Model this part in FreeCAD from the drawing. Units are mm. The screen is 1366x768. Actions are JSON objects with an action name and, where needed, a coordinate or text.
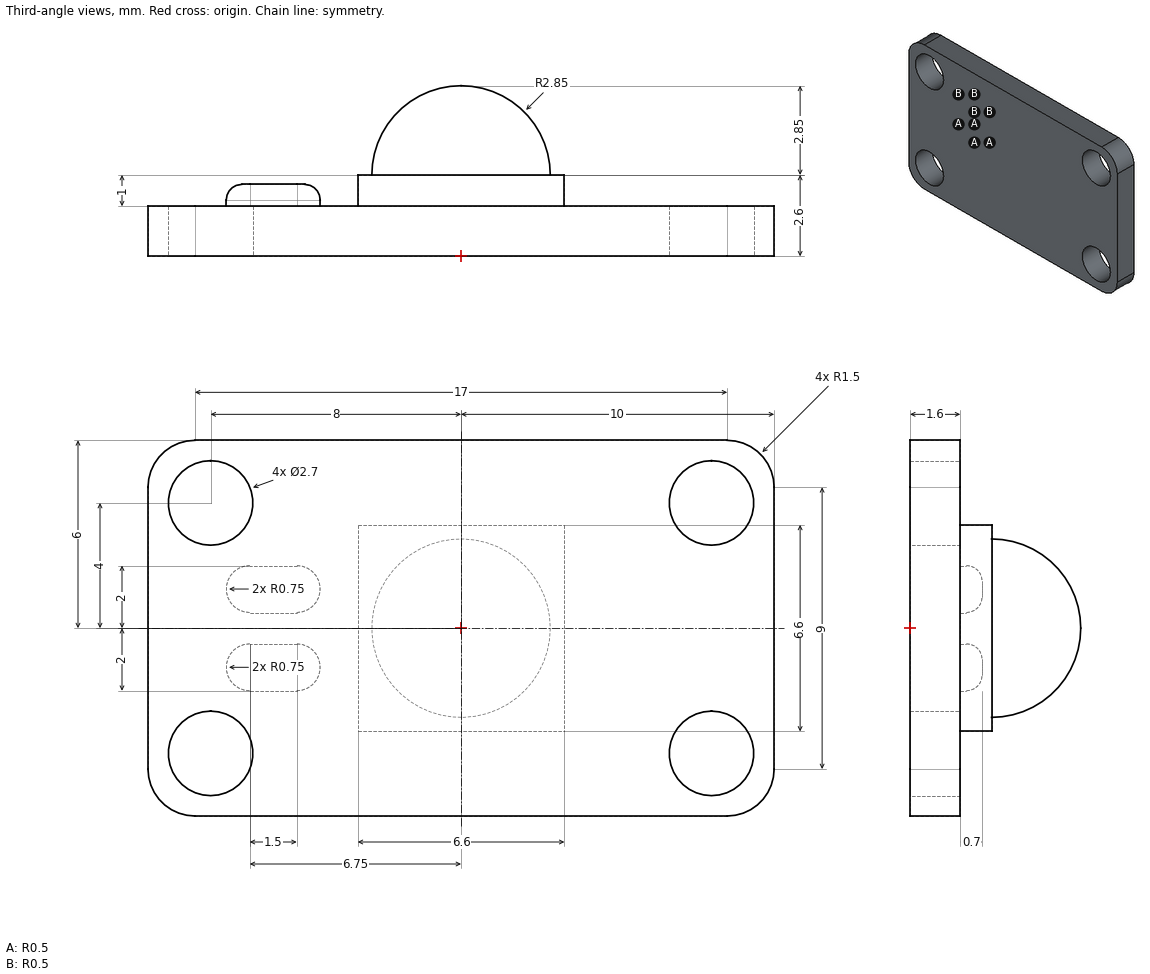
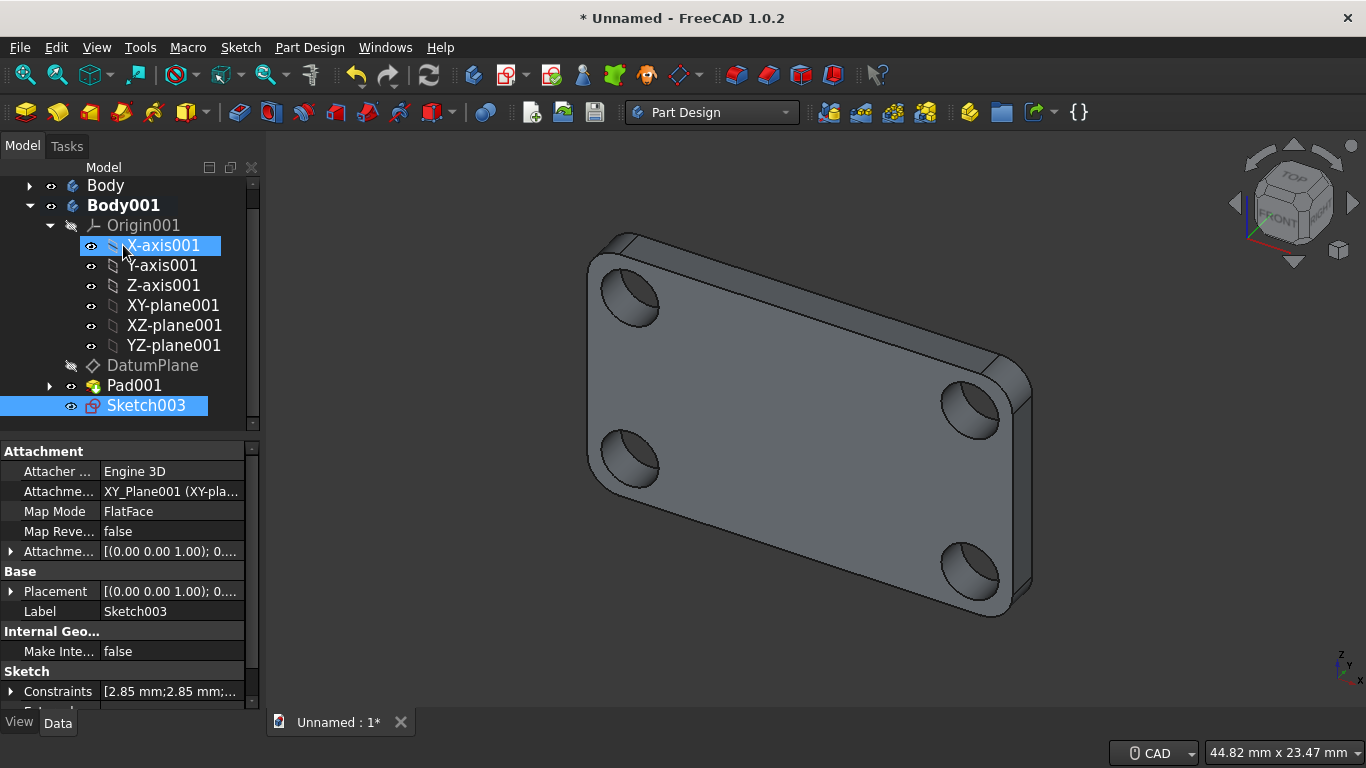
{"action": "left_click", "coordinate": [58, 112]}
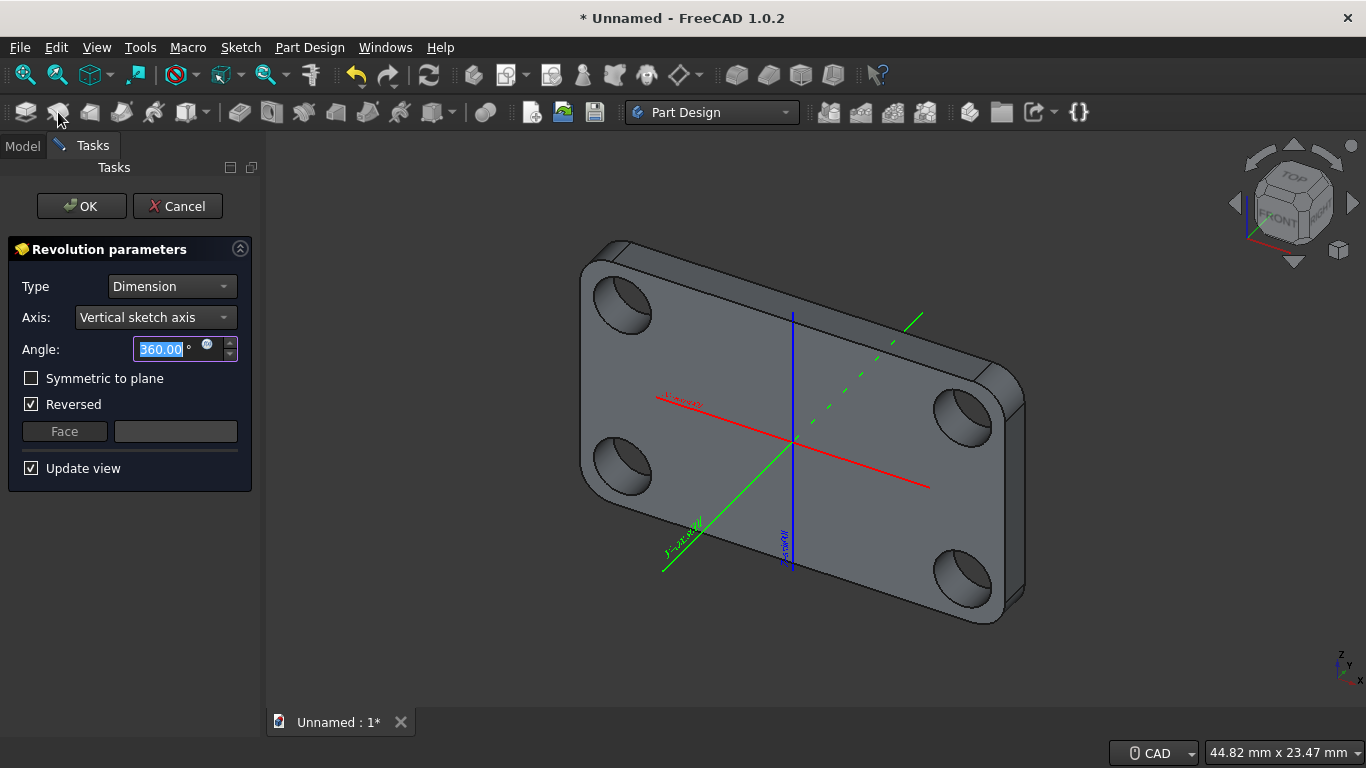
{"action": "left_click", "coordinate": [82, 206]}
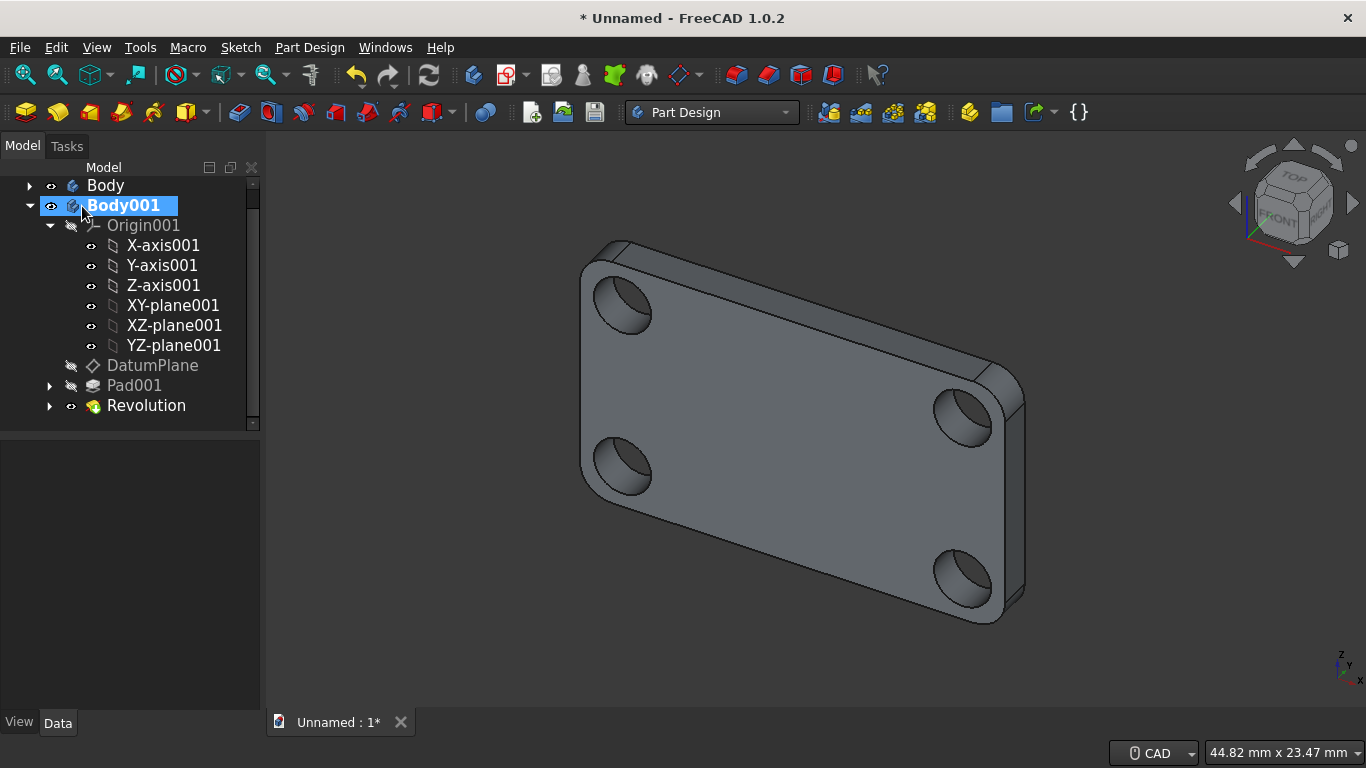
{"action": "key", "text": "v f"}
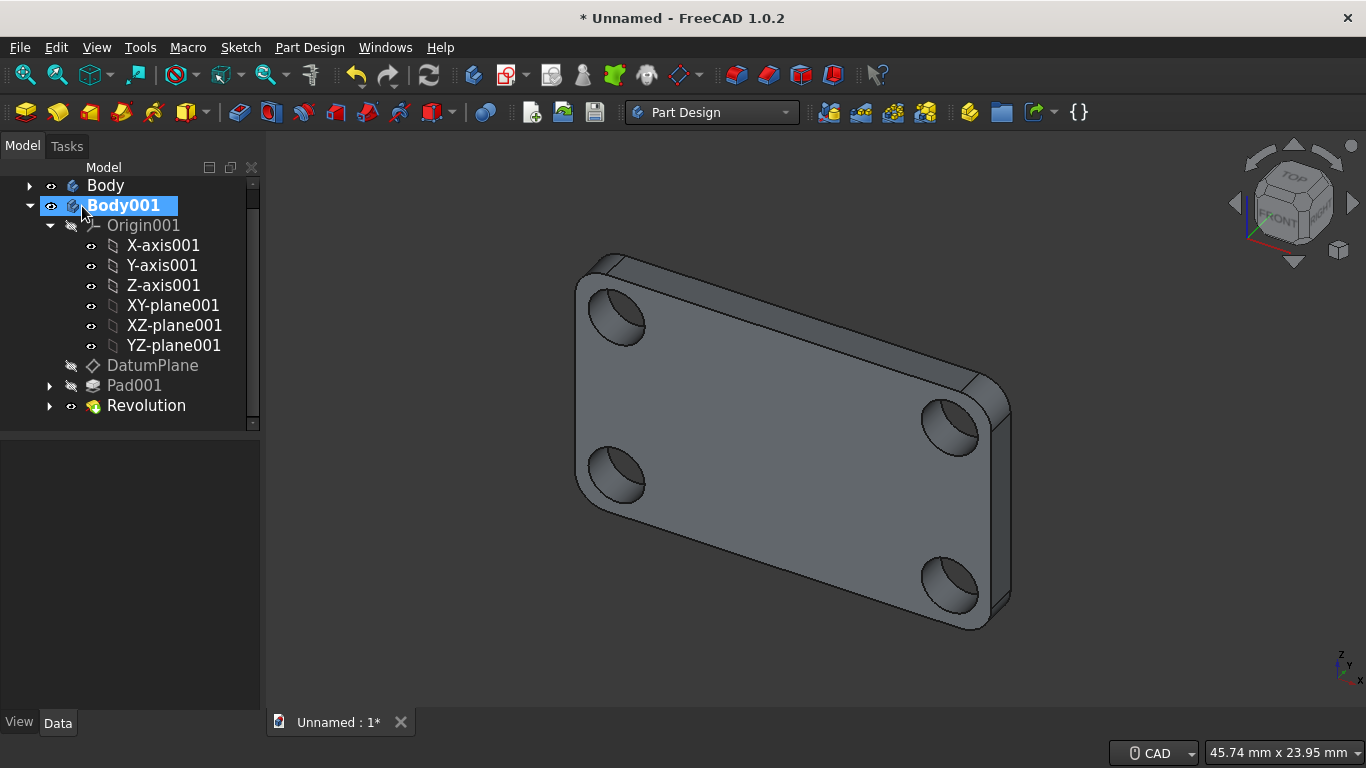
{"action": "left_click", "coordinate": [474, 76]}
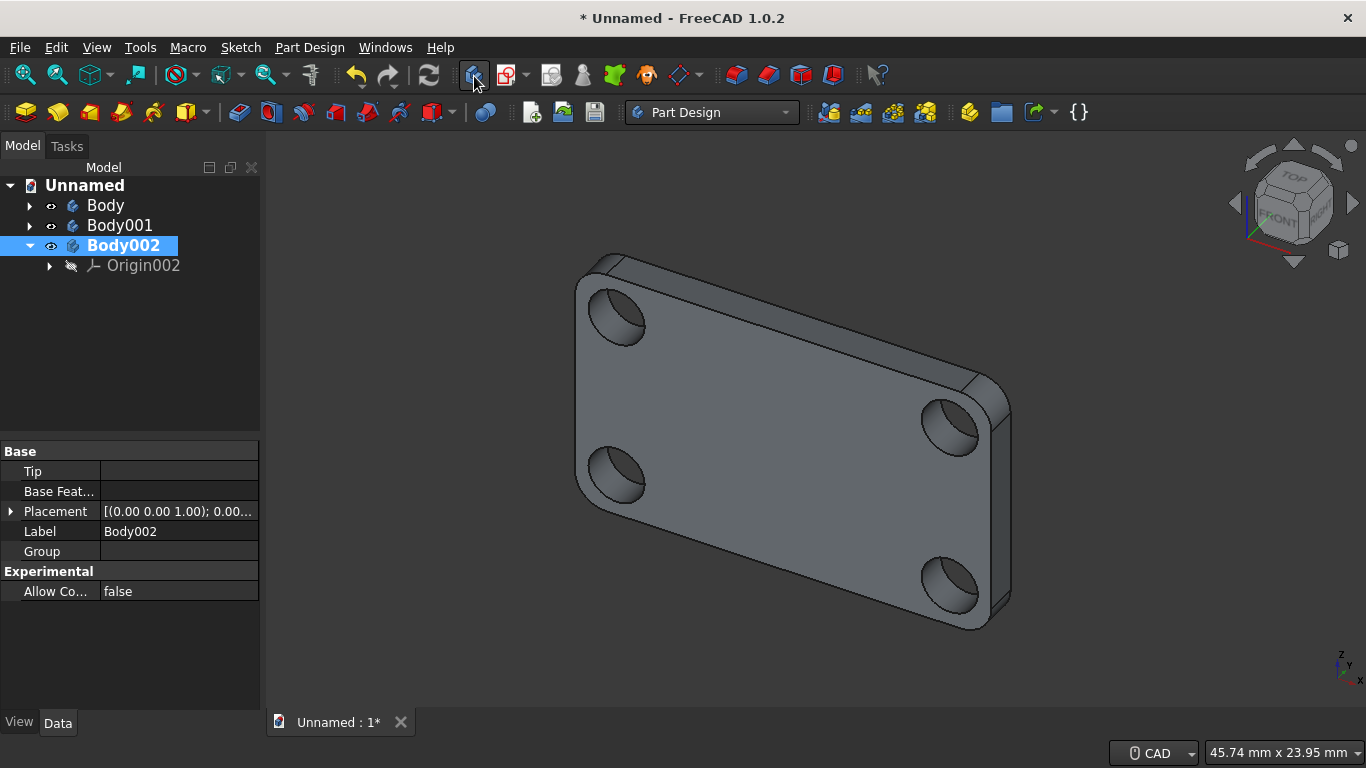
{"action": "left_click", "coordinate": [50, 266]}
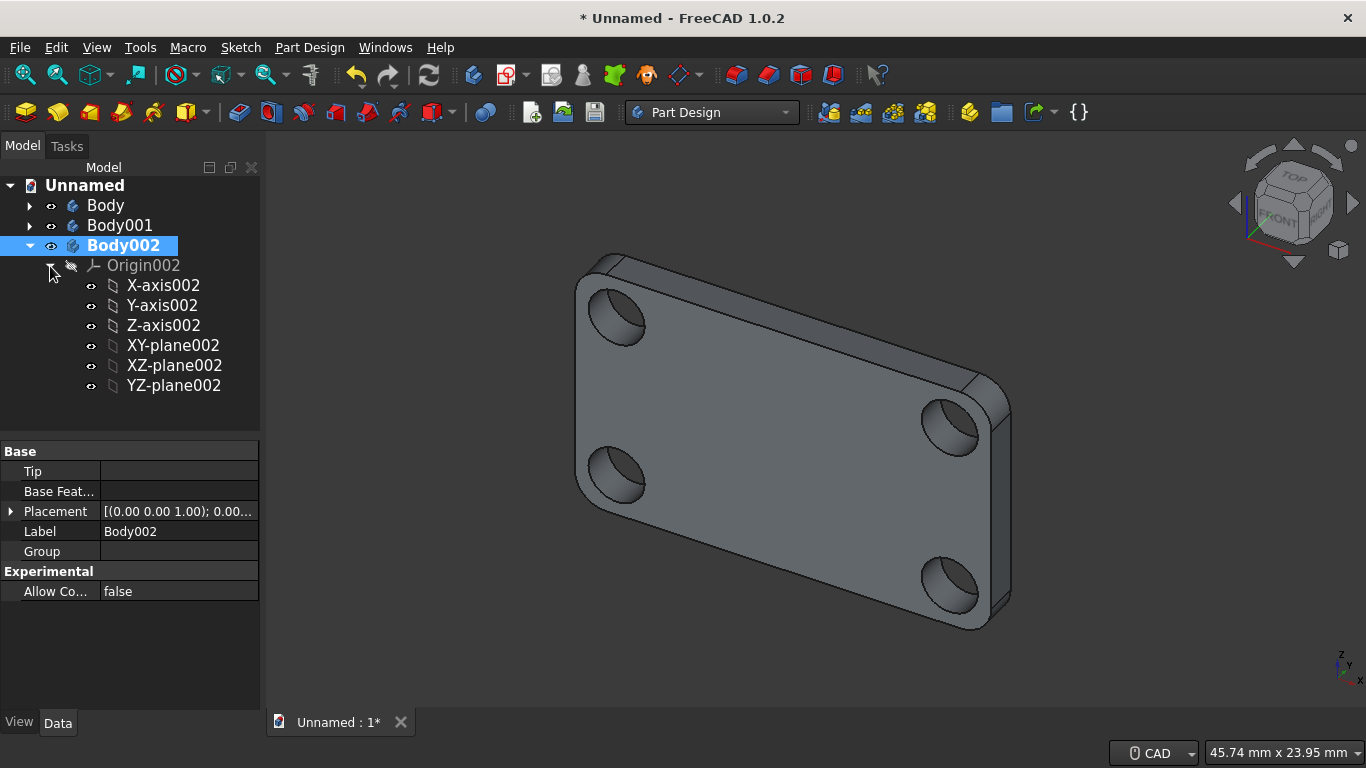
{"action": "left_click", "coordinate": [136, 366]}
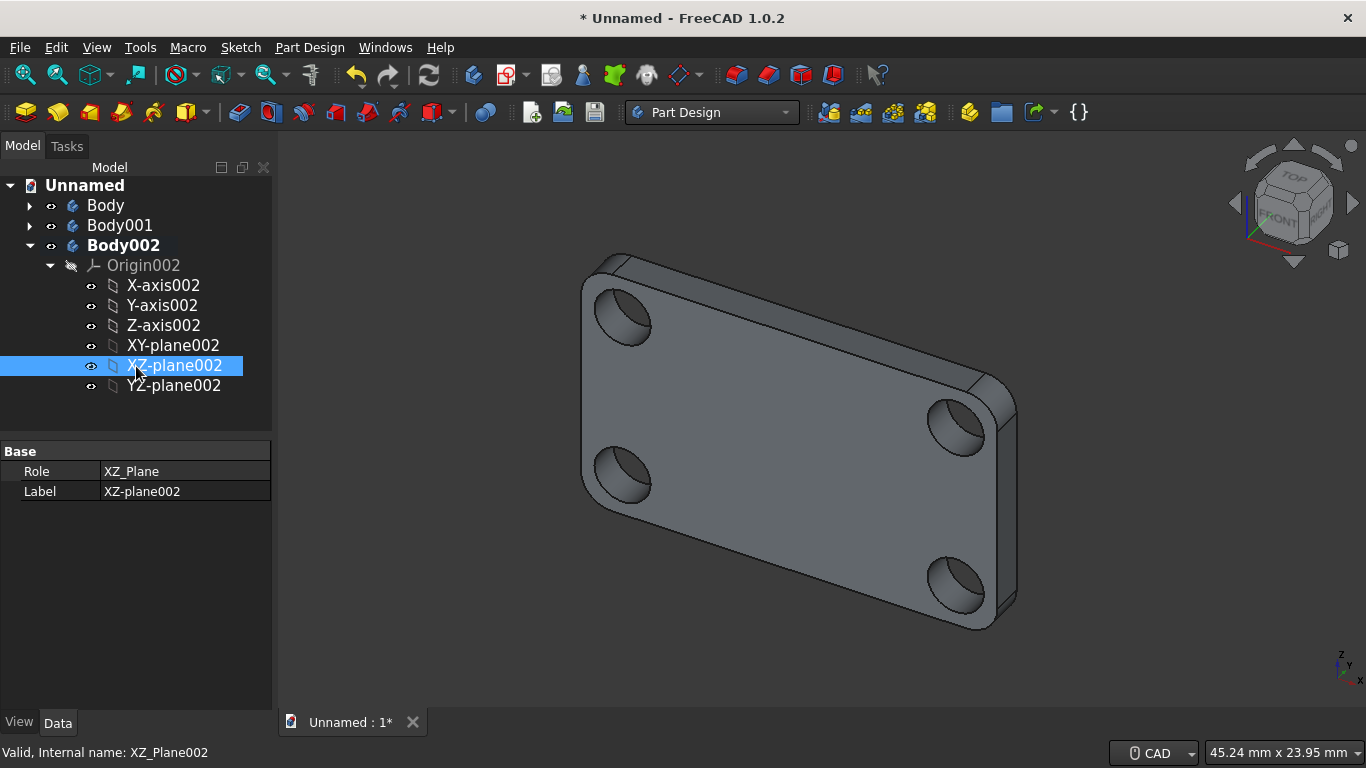
{"action": "left_click", "coordinate": [680, 76]}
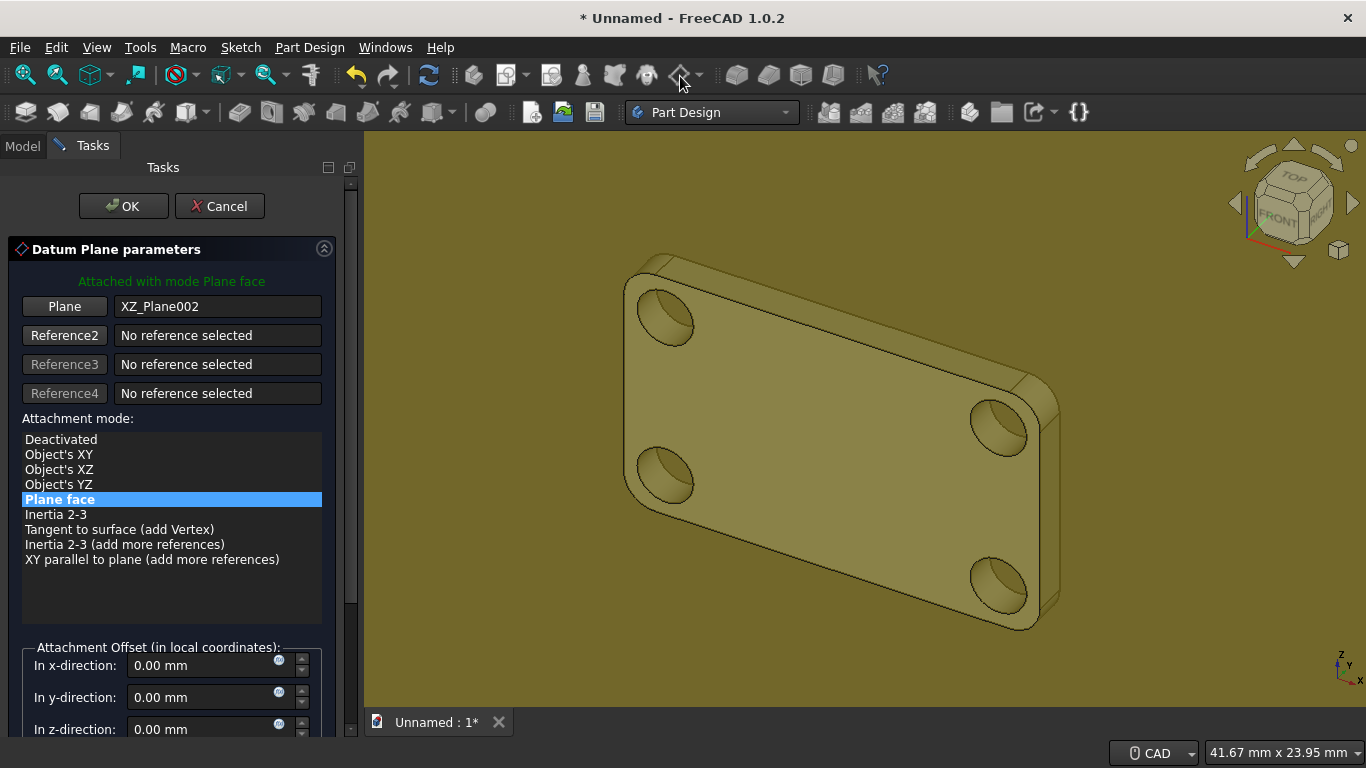
{"action": "scroll", "coordinate": [351, 456], "scroll_direction": "down", "scroll_amount": 2}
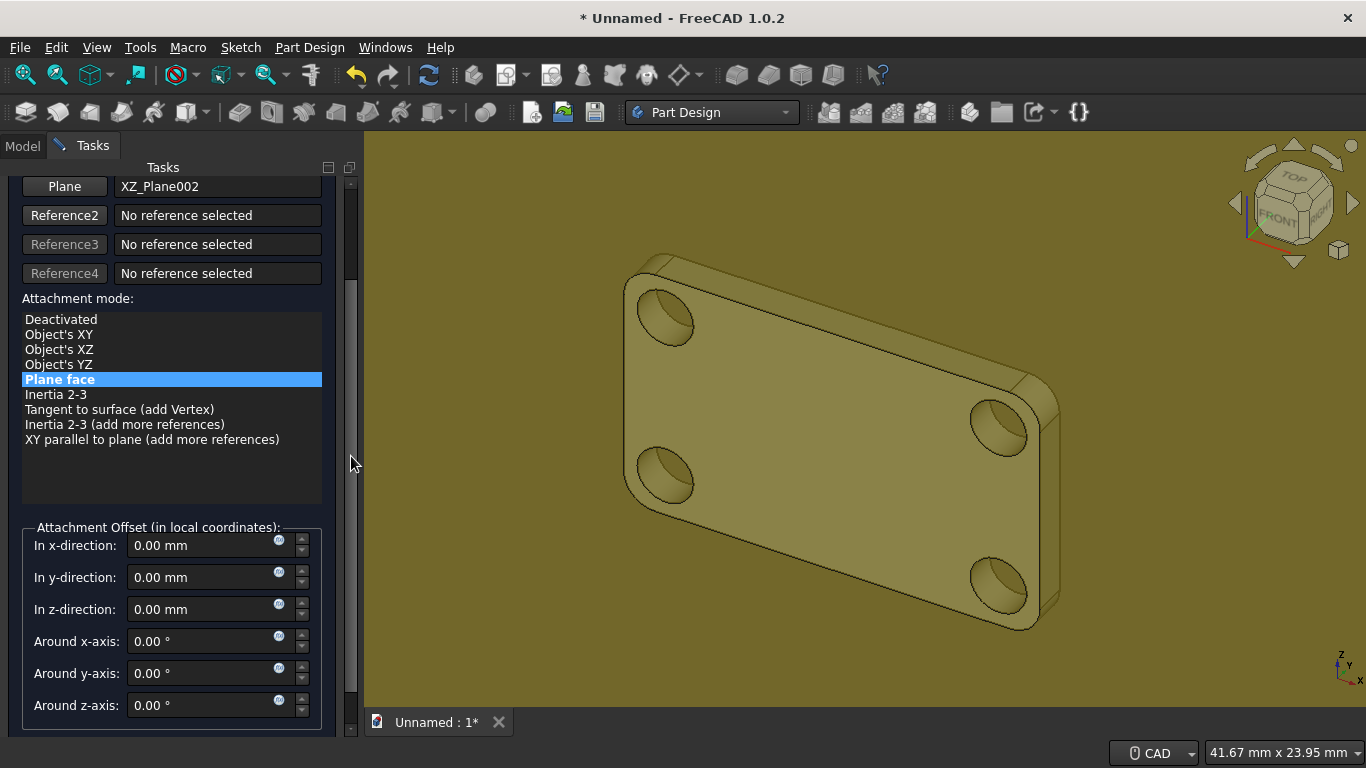
{"action": "triple_click", "coordinate": [210, 609]}